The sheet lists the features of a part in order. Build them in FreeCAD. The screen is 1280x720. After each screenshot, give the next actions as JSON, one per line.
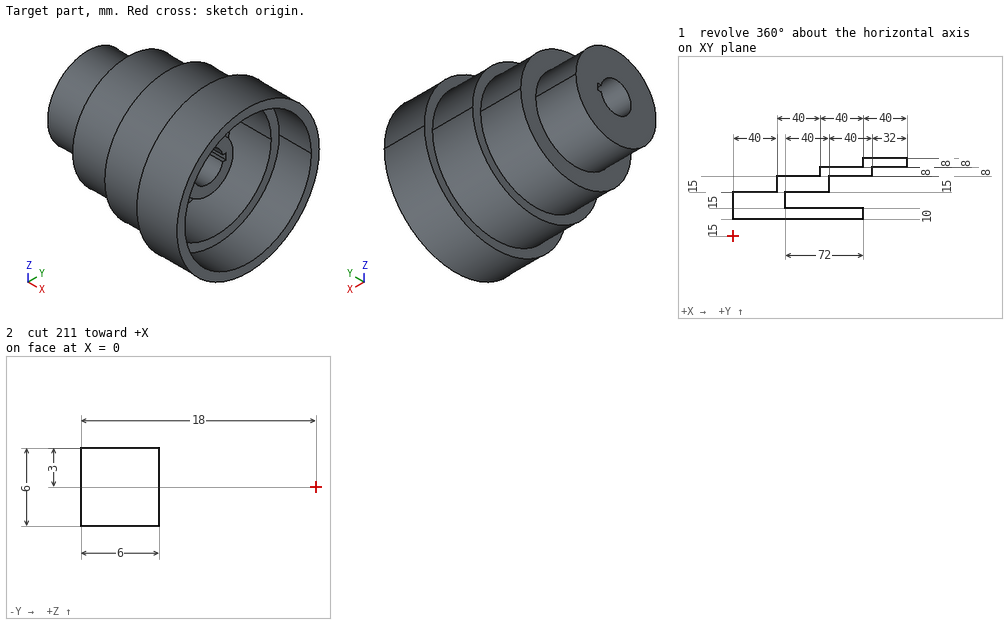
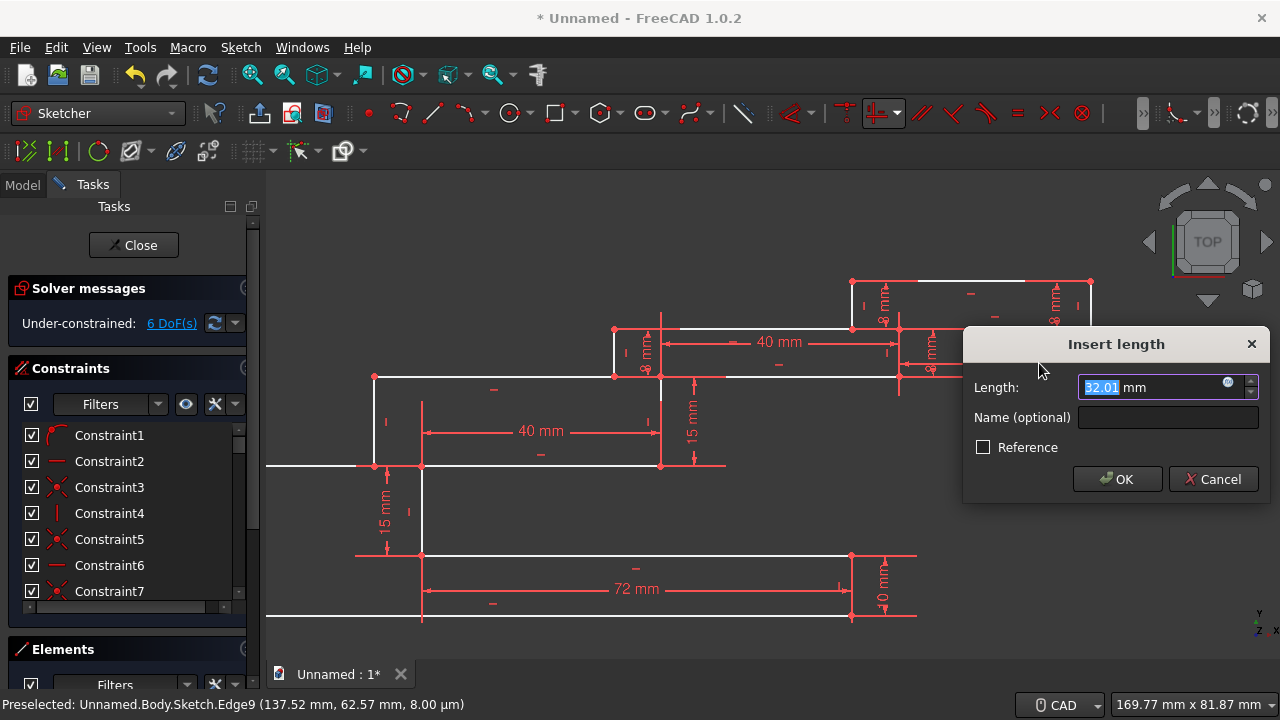
{"action": "type", "text": "32"}
{"action": "key", "text": "Return"}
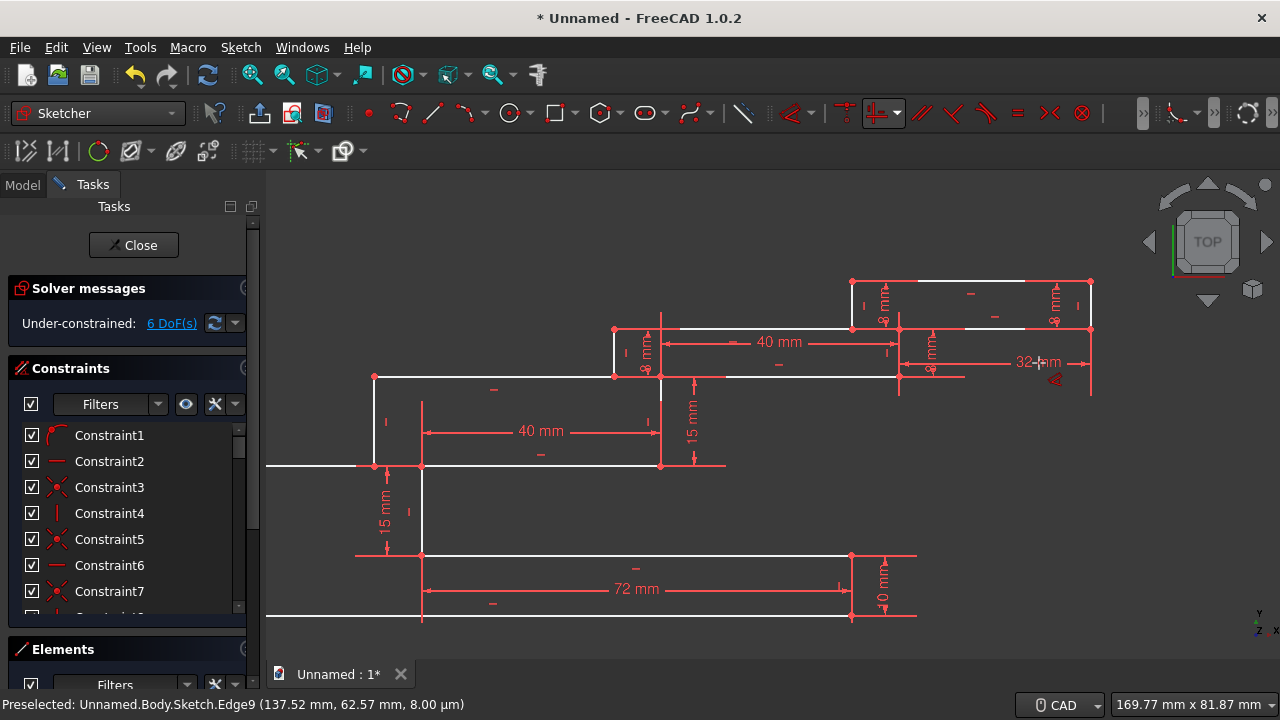
{"action": "left_click", "coordinate": [1019, 281]}
{"action": "left_click", "coordinate": [972, 247]}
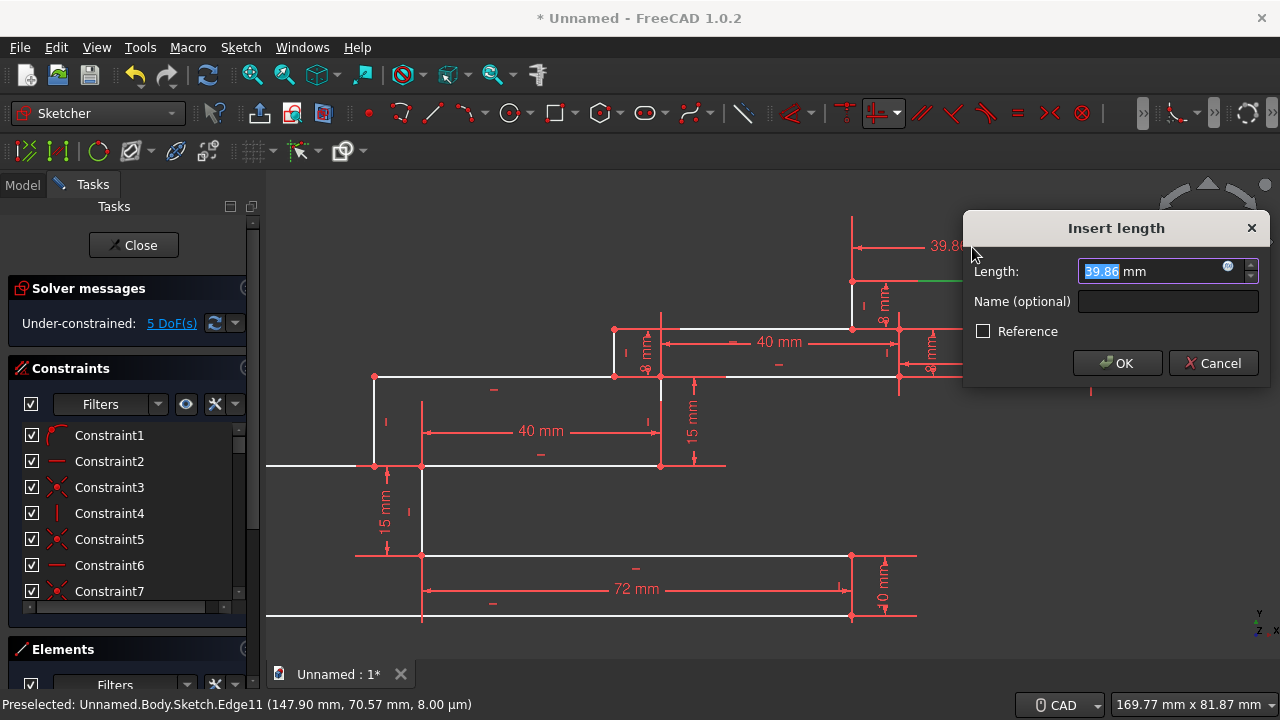
{"action": "type", "text": "40"}
{"action": "key", "text": "Return"}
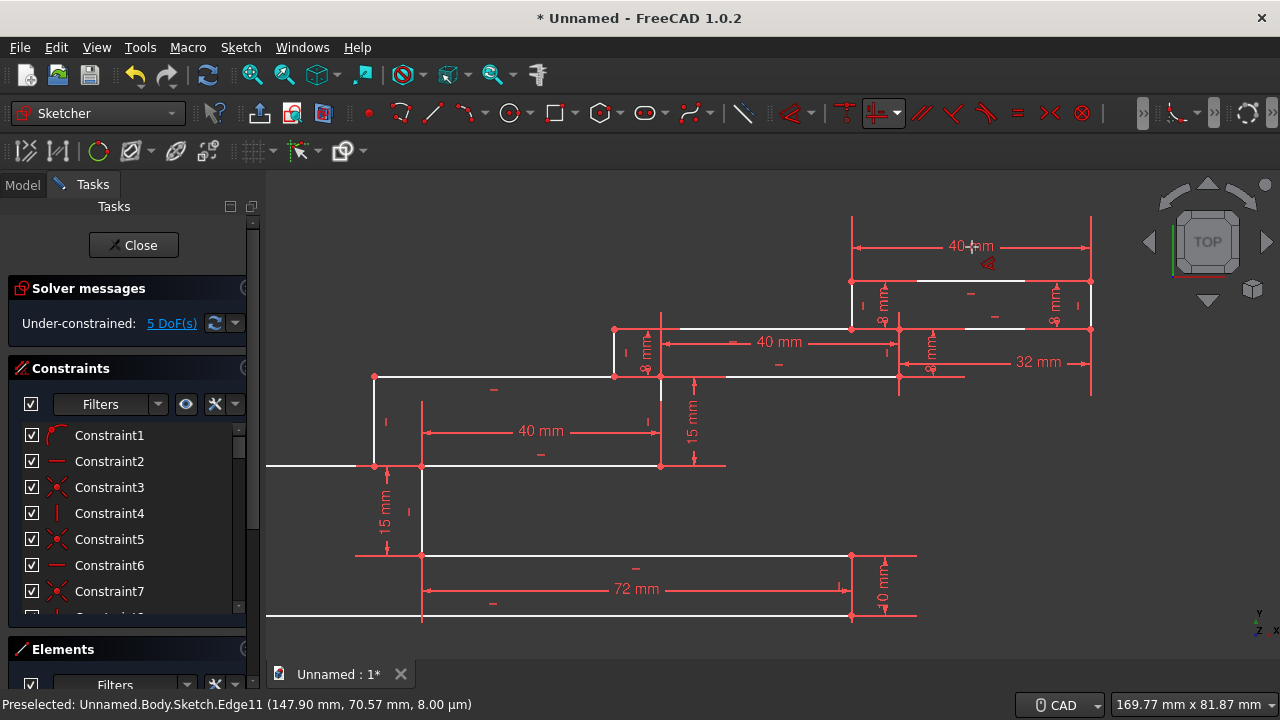
{"action": "left_click", "coordinate": [780, 329]}
{"action": "left_click", "coordinate": [733, 295]}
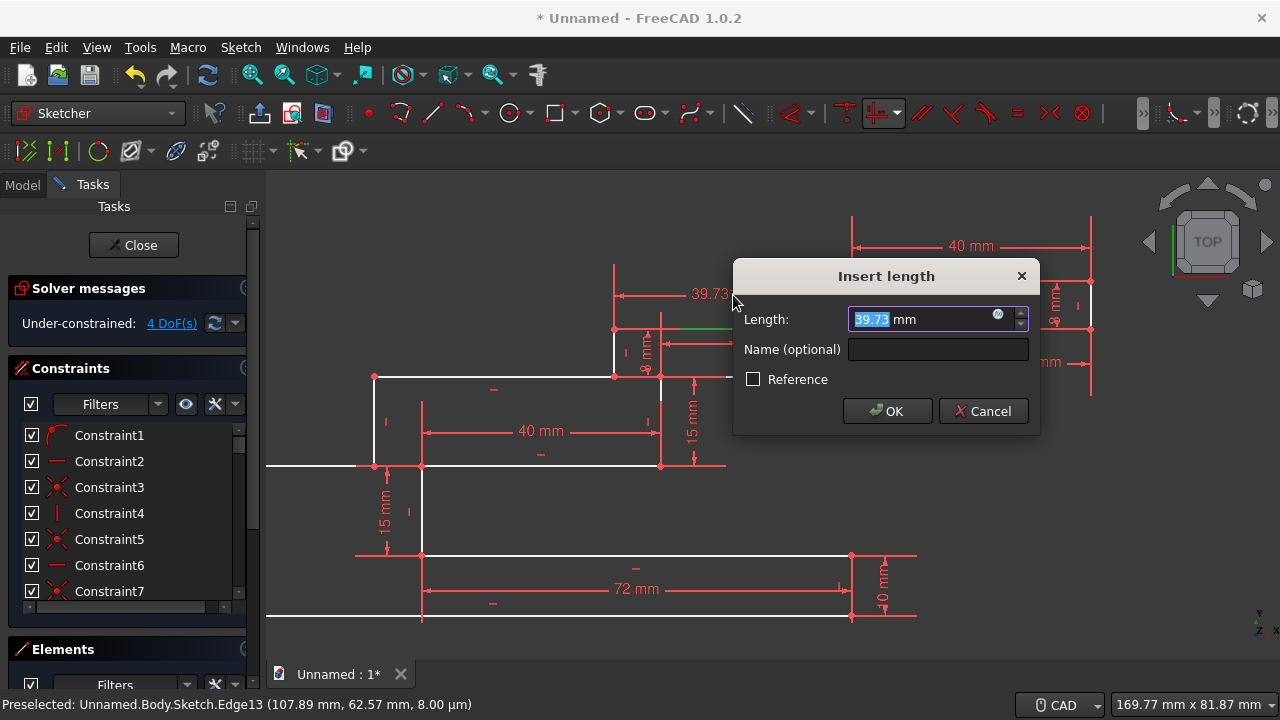
{"action": "type", "text": "40"}
{"action": "key", "text": "Return"}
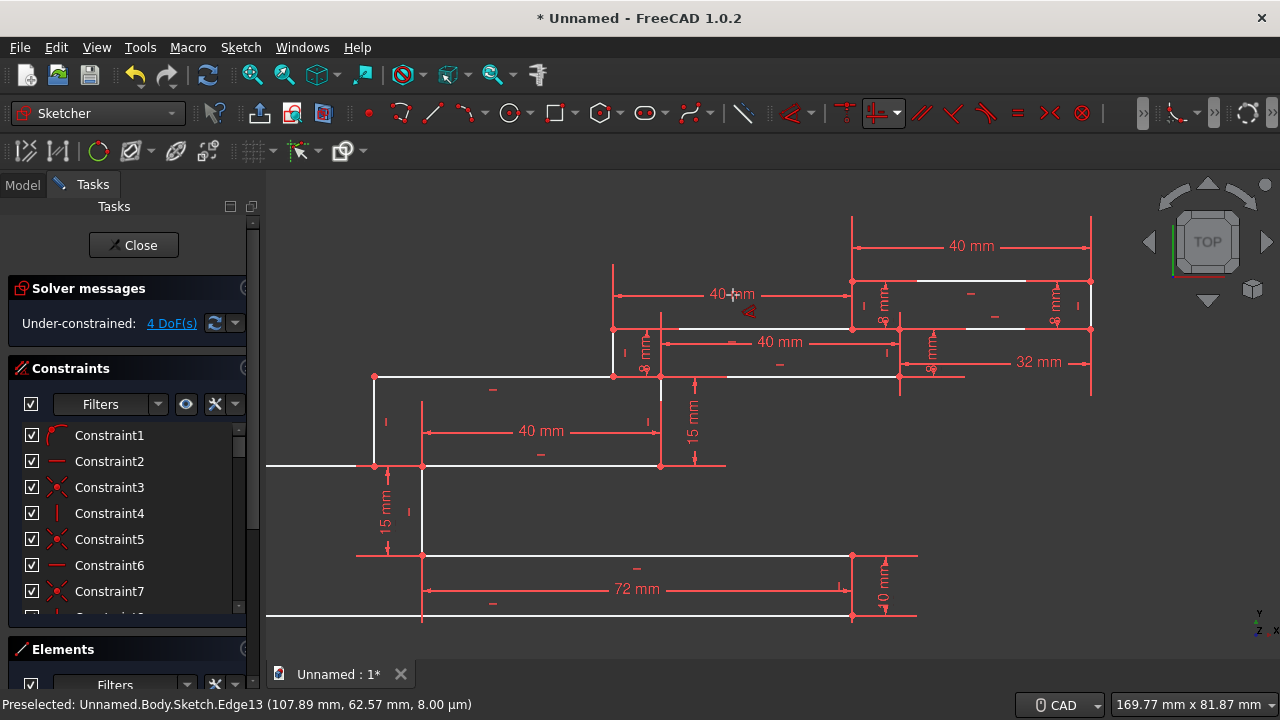
{"action": "left_click", "coordinate": [541, 377]}
{"action": "left_click", "coordinate": [494, 343]}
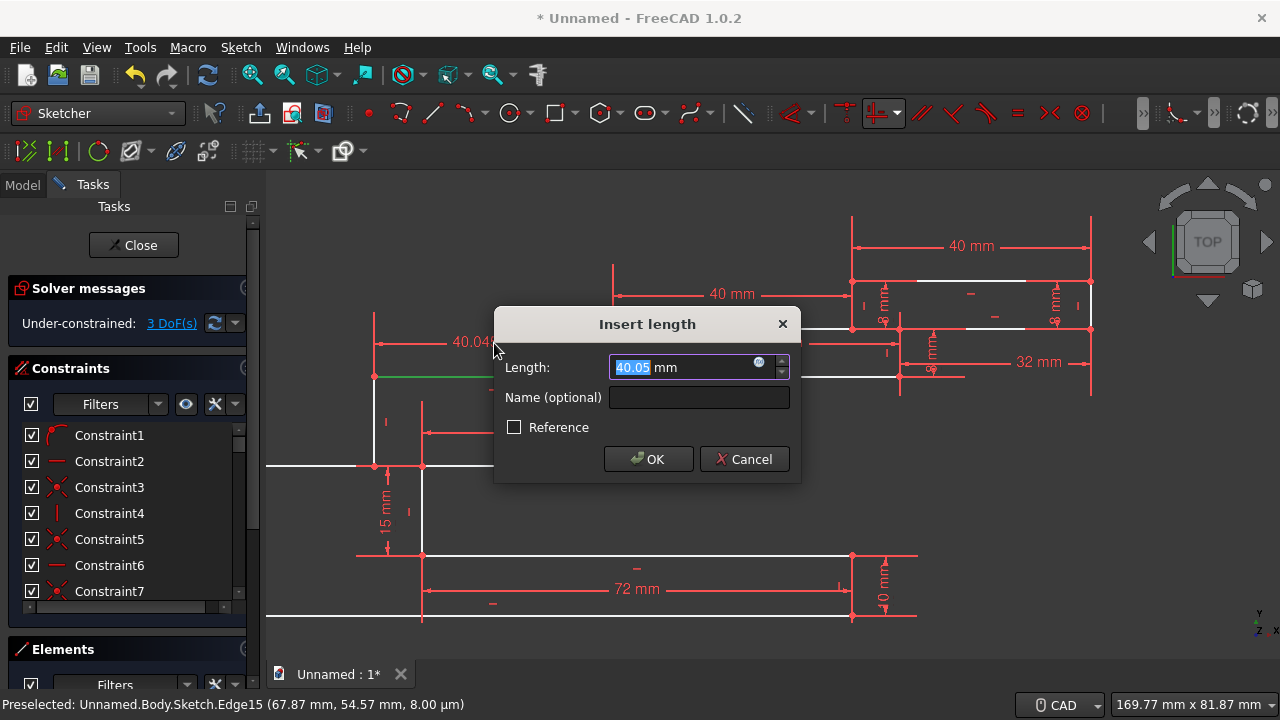
{"action": "type", "text": "40"}
{"action": "key", "text": "Return"}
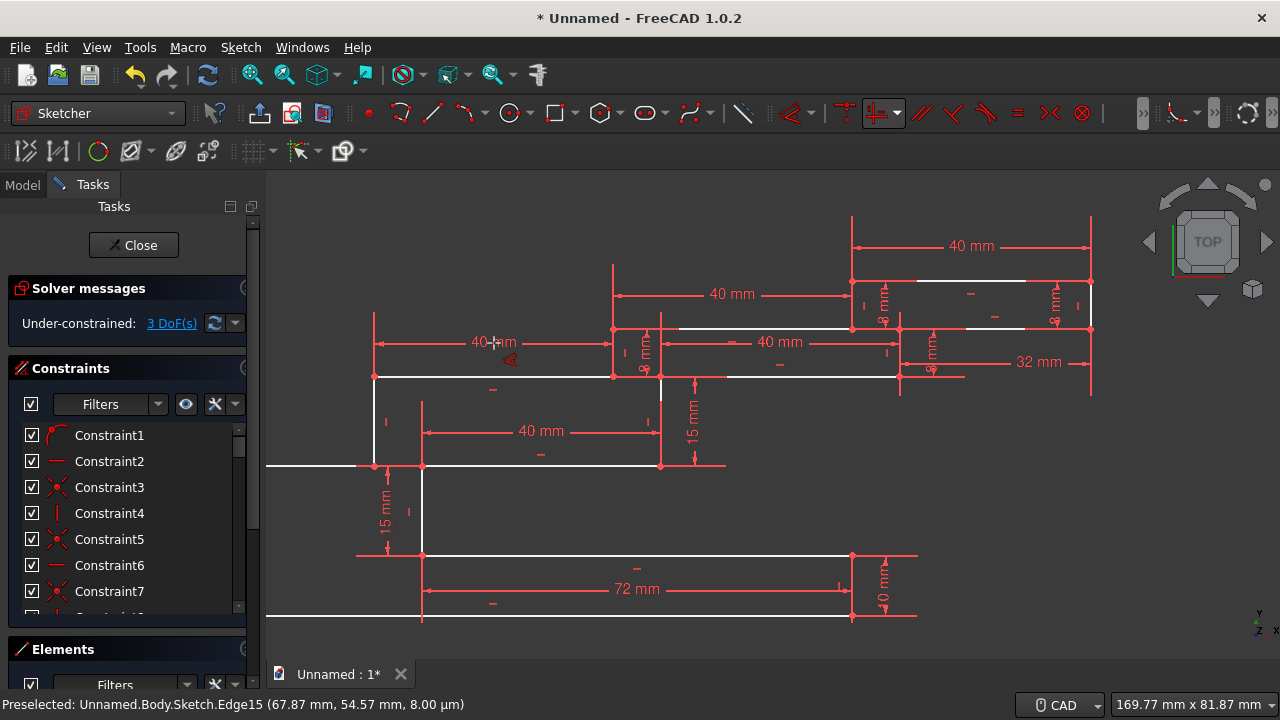
{"action": "left_click", "coordinate": [374, 404]}
{"action": "left_click", "coordinate": [340, 421]}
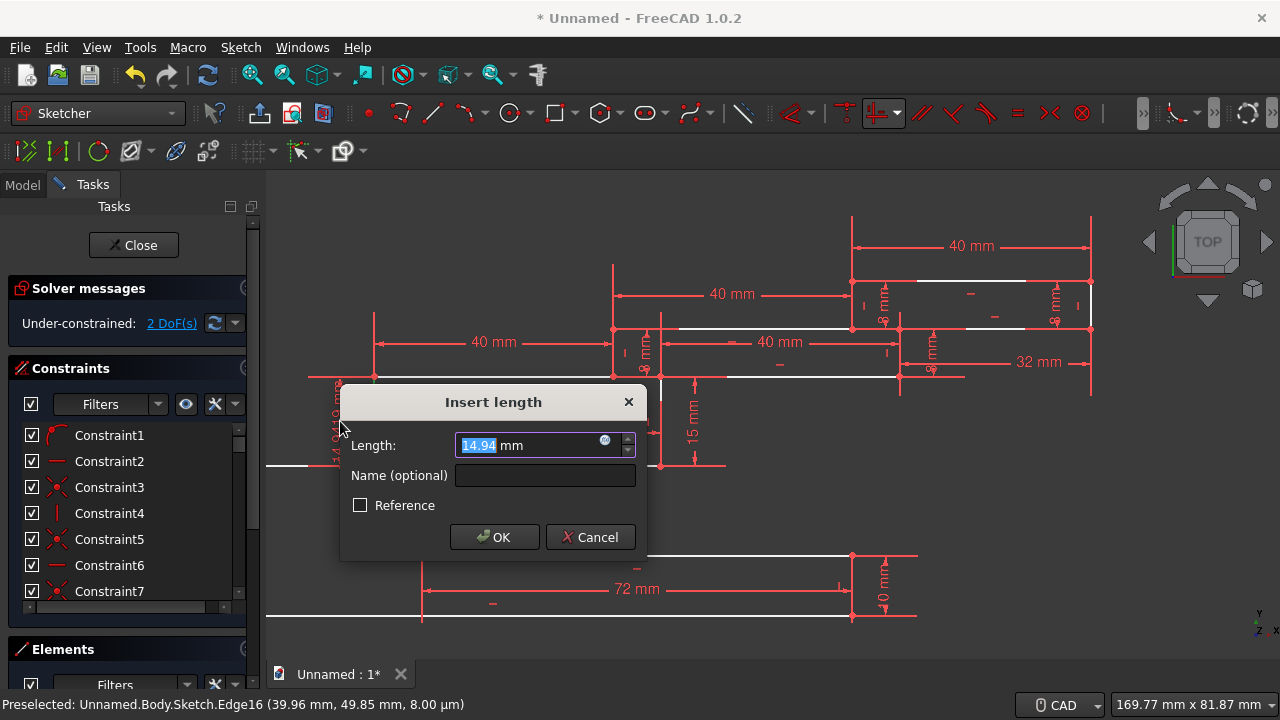
{"action": "type", "text": "15"}
{"action": "key", "text": "Return"}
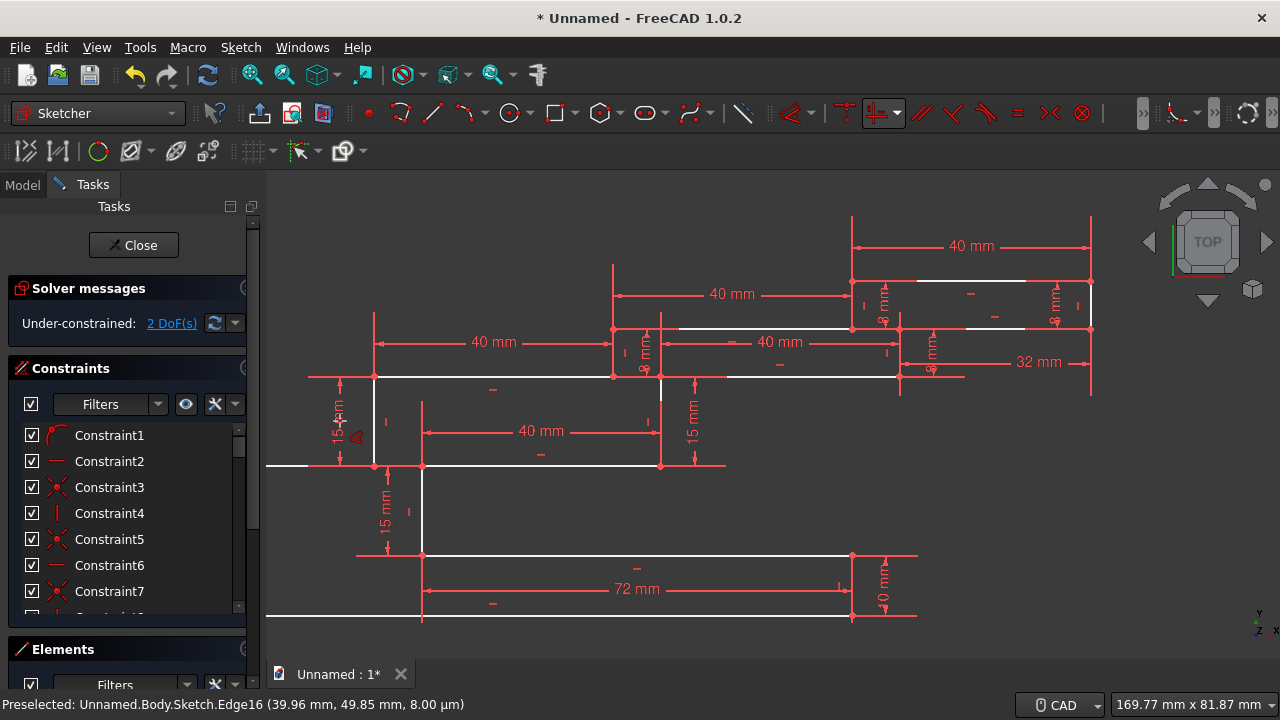
{"action": "left_click", "coordinate": [303, 466]}
{"action": "left_click", "coordinate": [316, 500]}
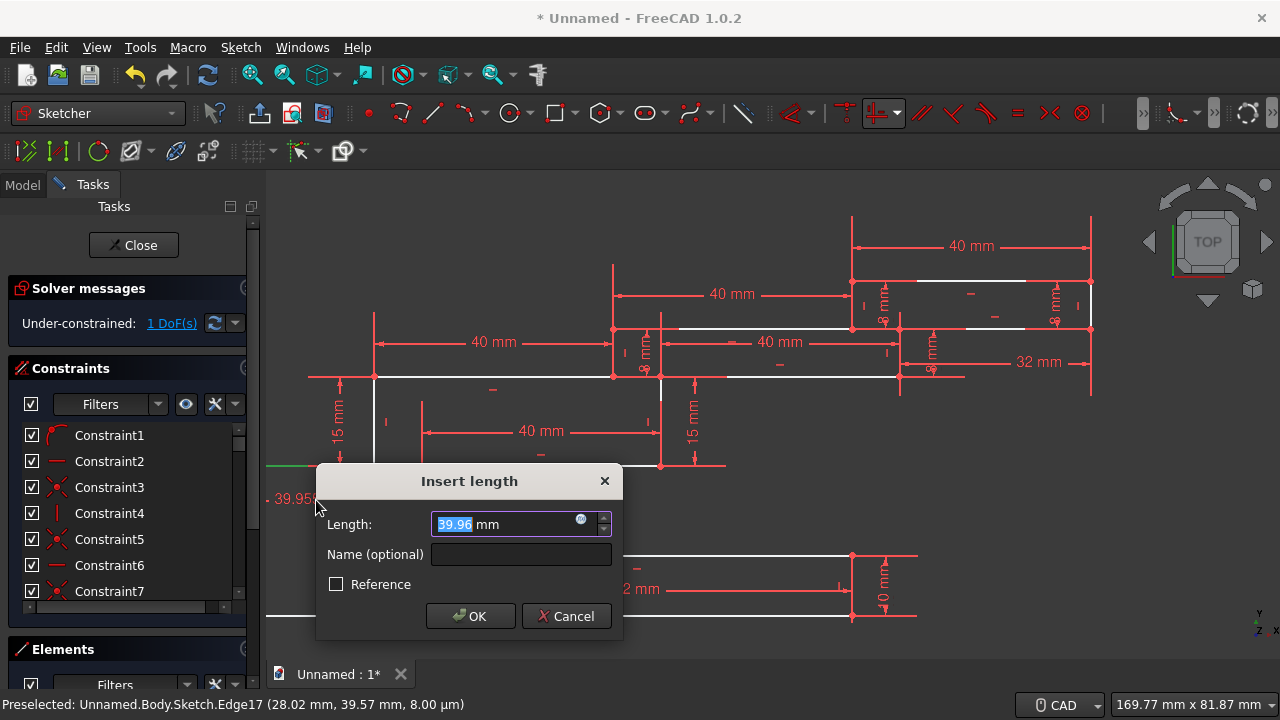
{"action": "type", "text": "40"}
{"action": "key", "text": "Return"}